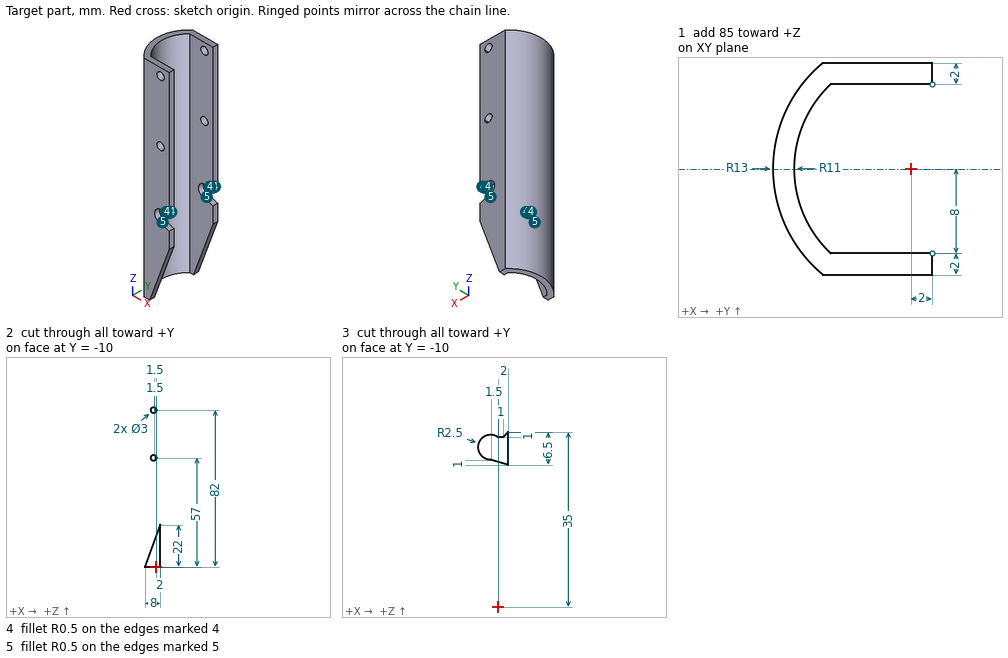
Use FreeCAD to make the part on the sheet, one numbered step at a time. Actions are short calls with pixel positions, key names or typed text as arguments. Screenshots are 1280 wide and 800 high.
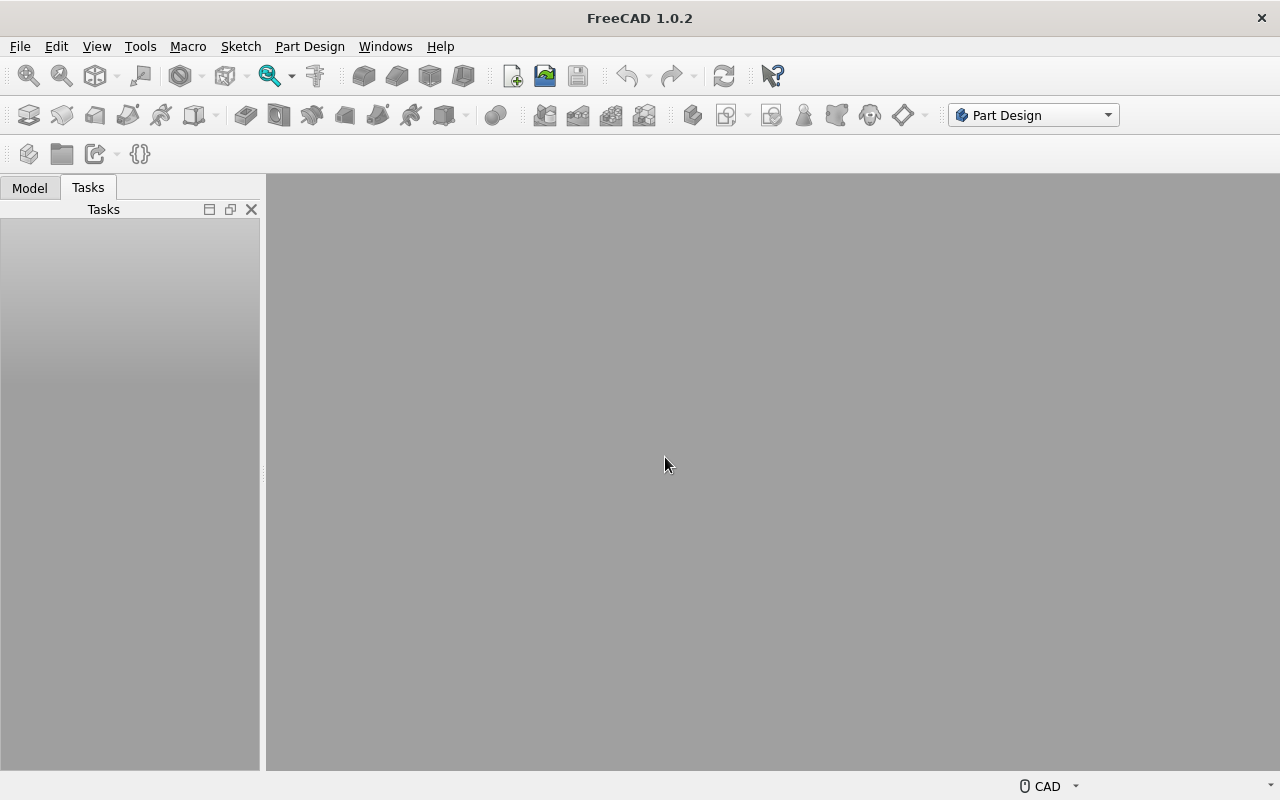
click(512, 76)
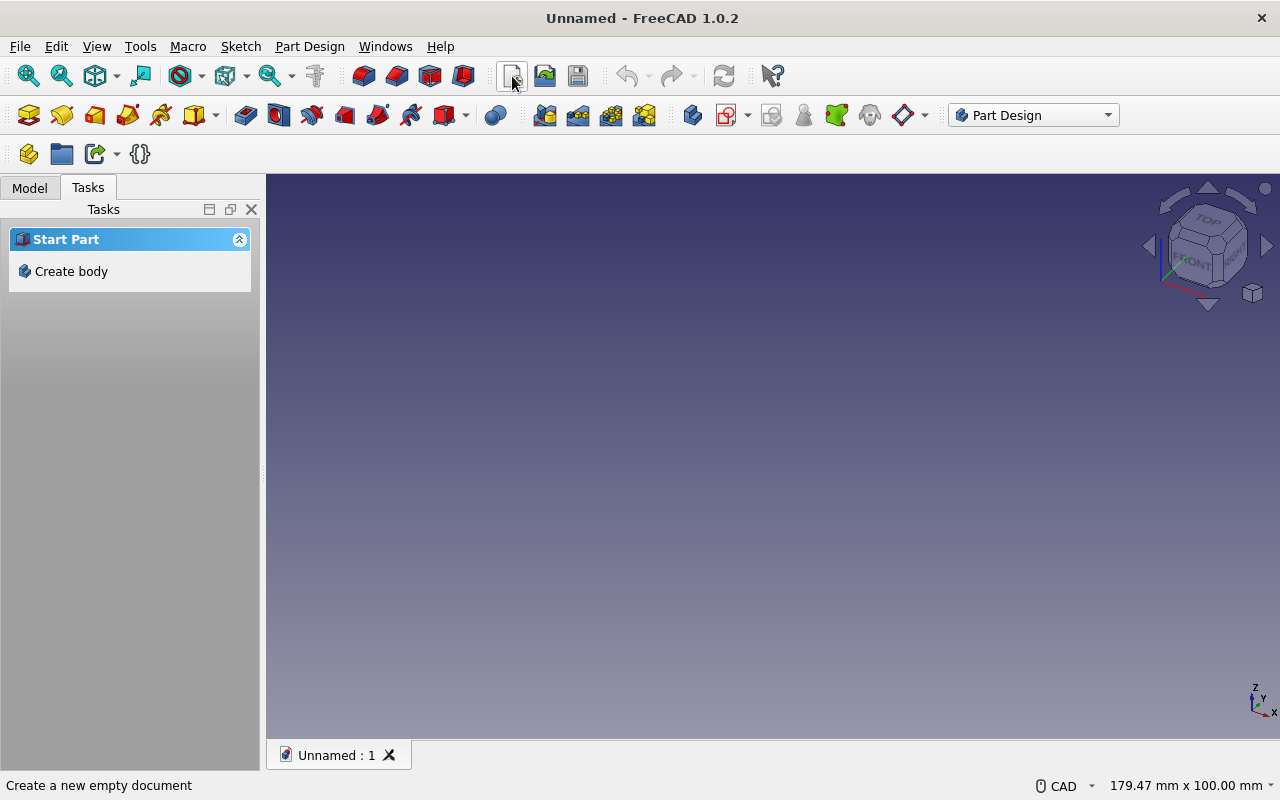
click(726, 116)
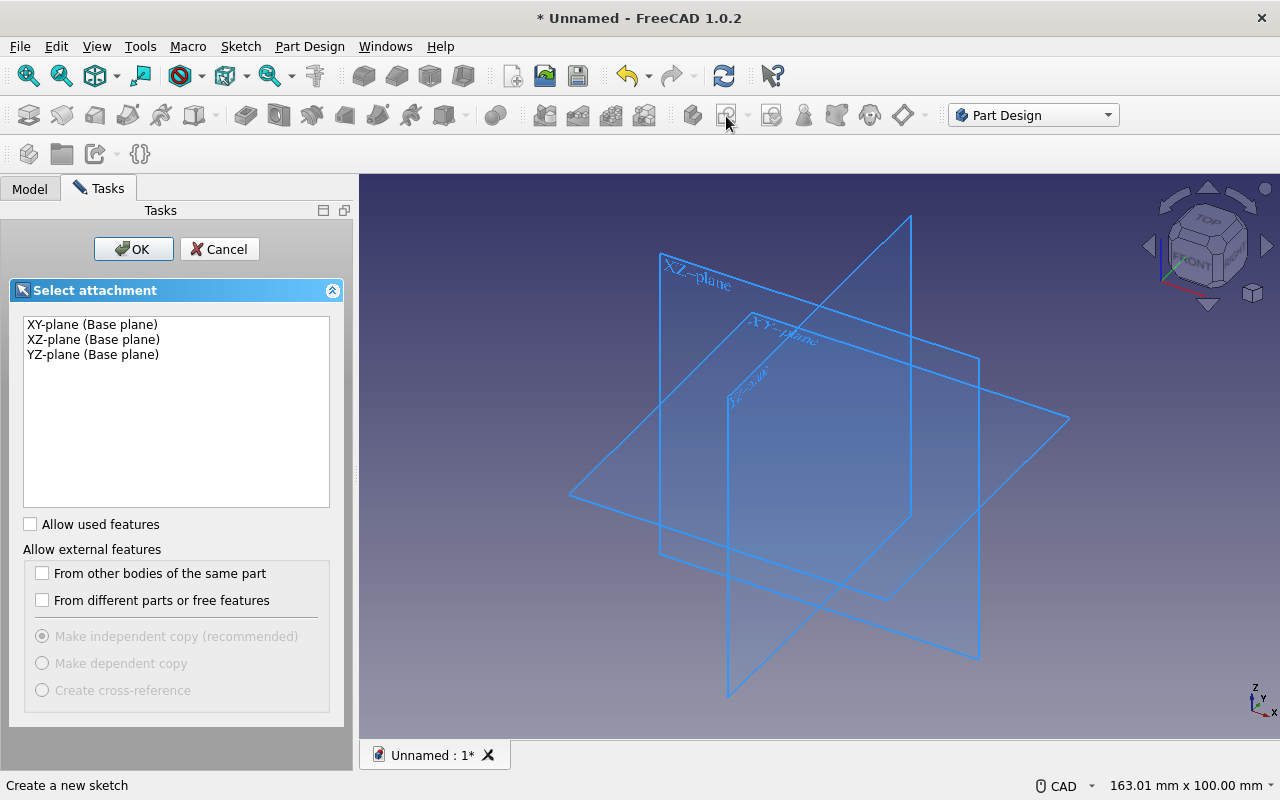
click(84, 324)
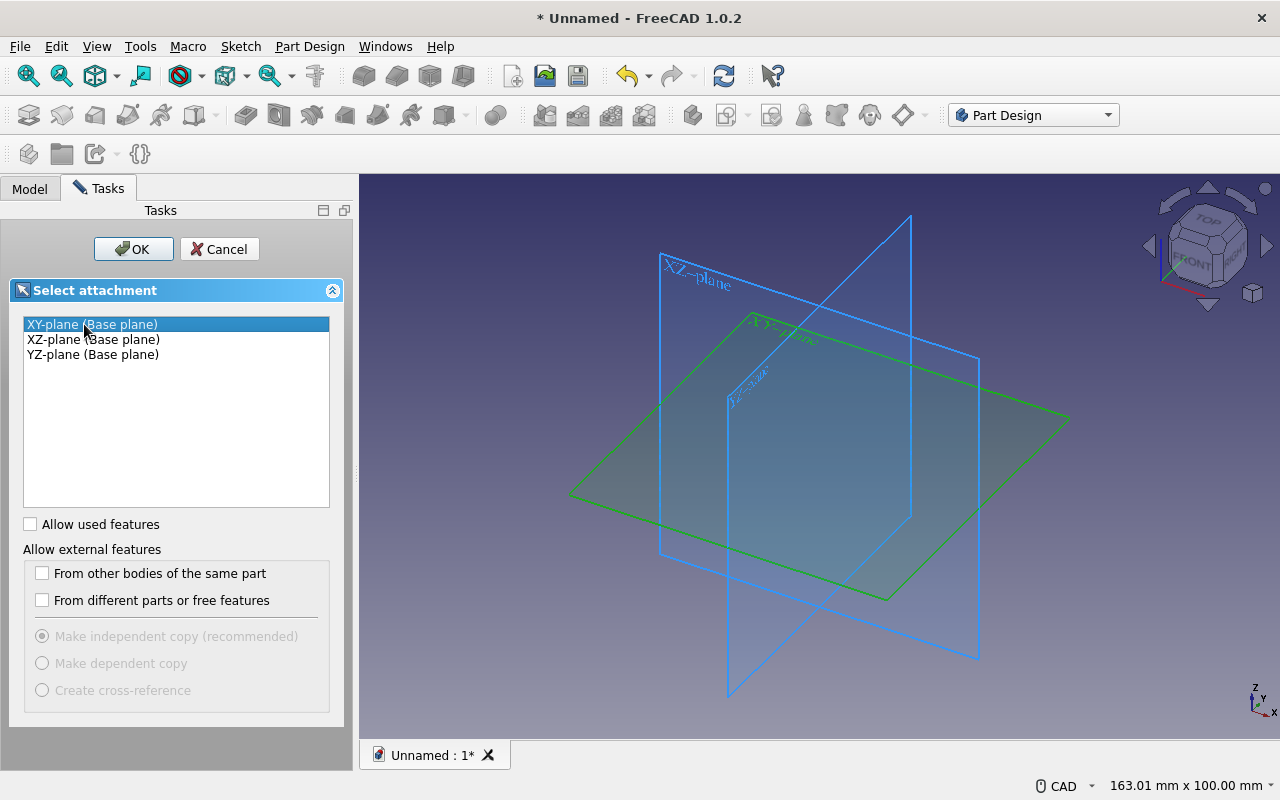
click(134, 249)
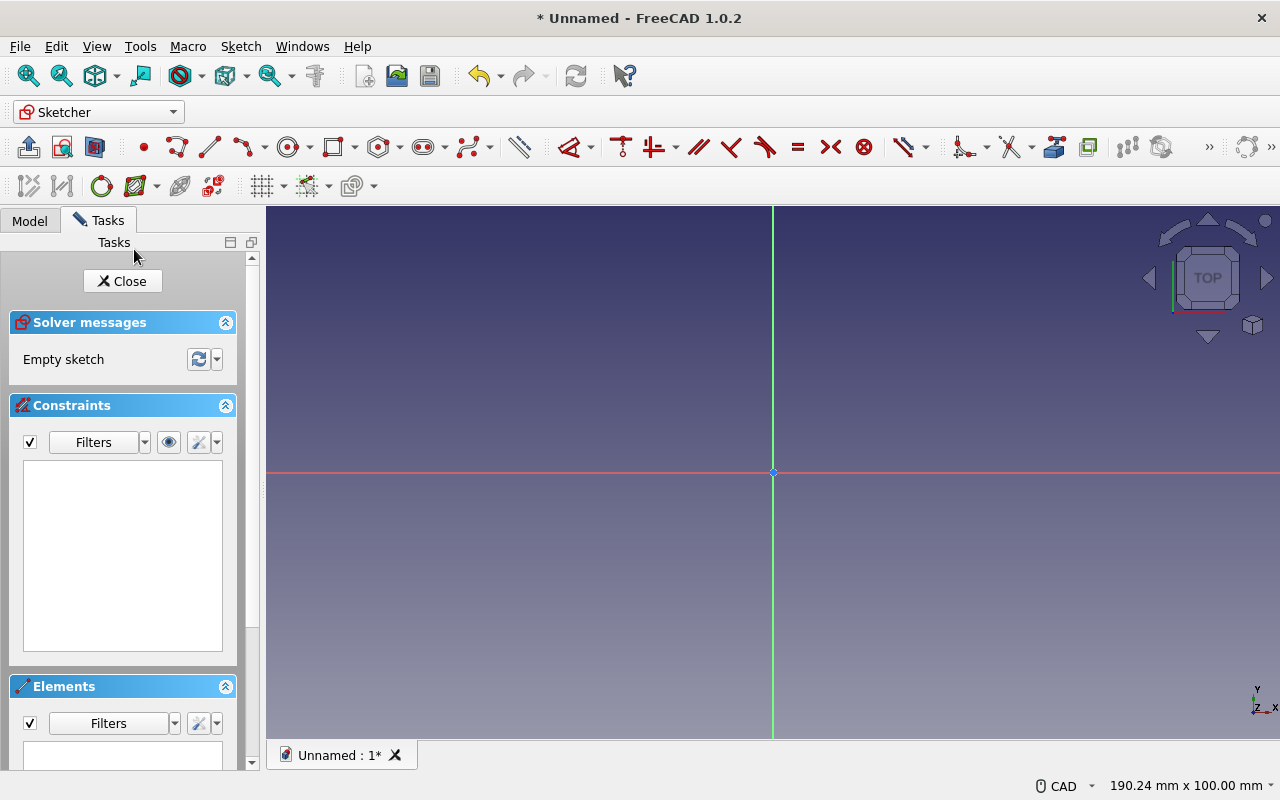
scroll(761, 472, up, 6)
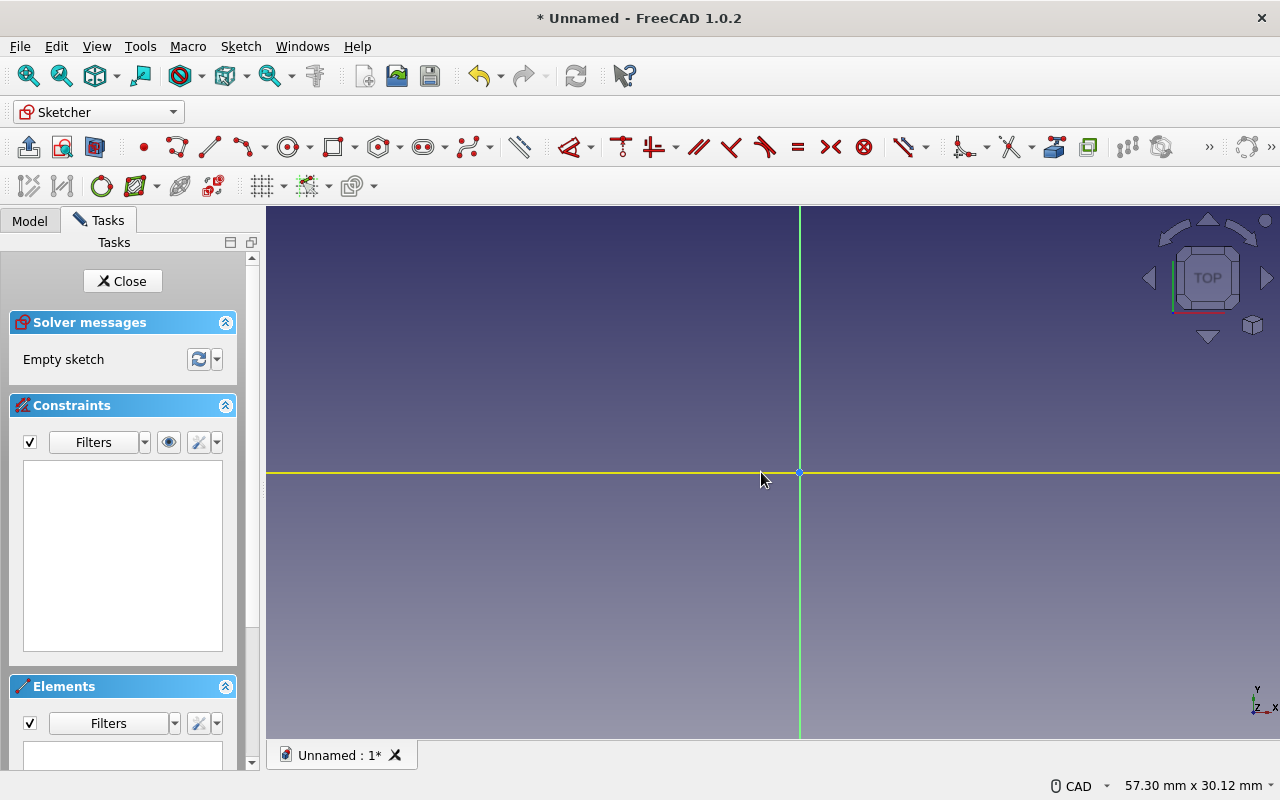
click(177, 148)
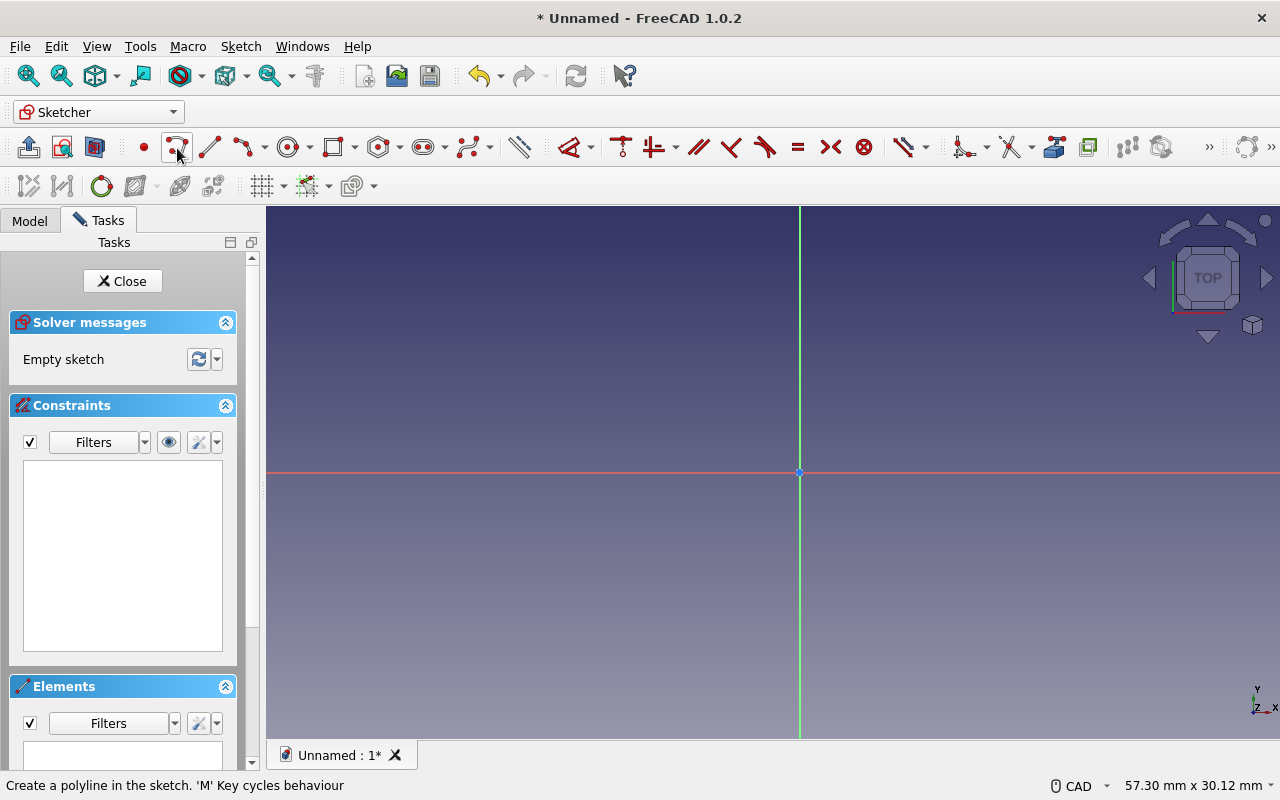
click(653, 649)
click(835, 649)
click(835, 614)
click(666, 614)
right_click(666, 614)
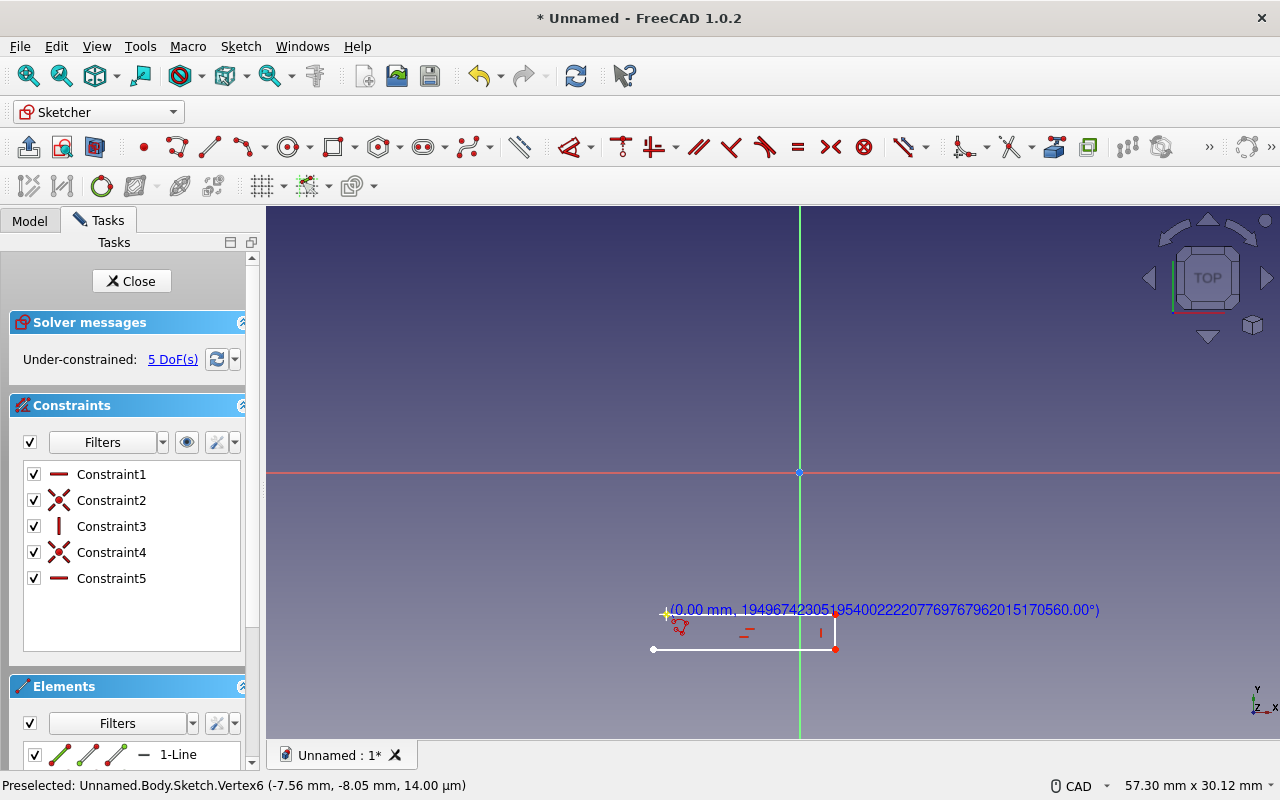
click(666, 331)
click(835, 331)
click(835, 296)
click(653, 296)
right_click(653, 296)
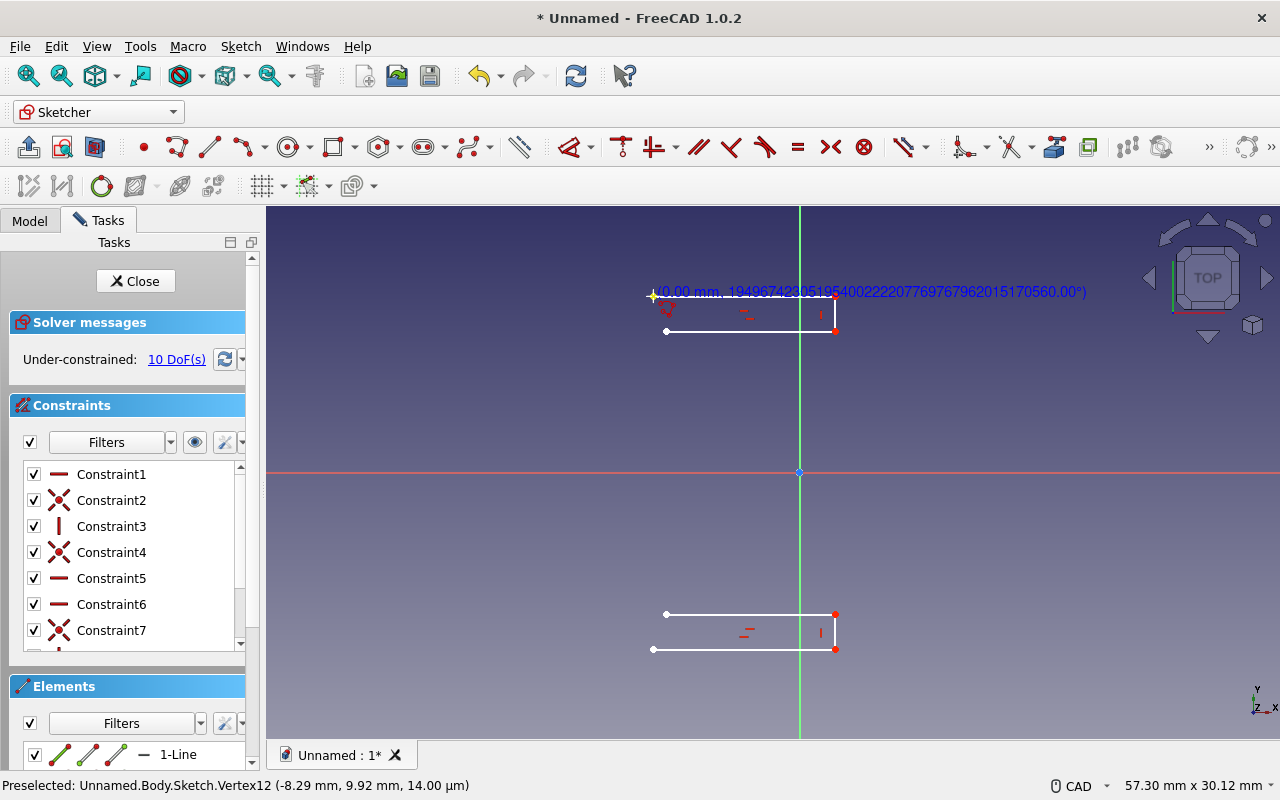
key(g)
key(3)
key(a)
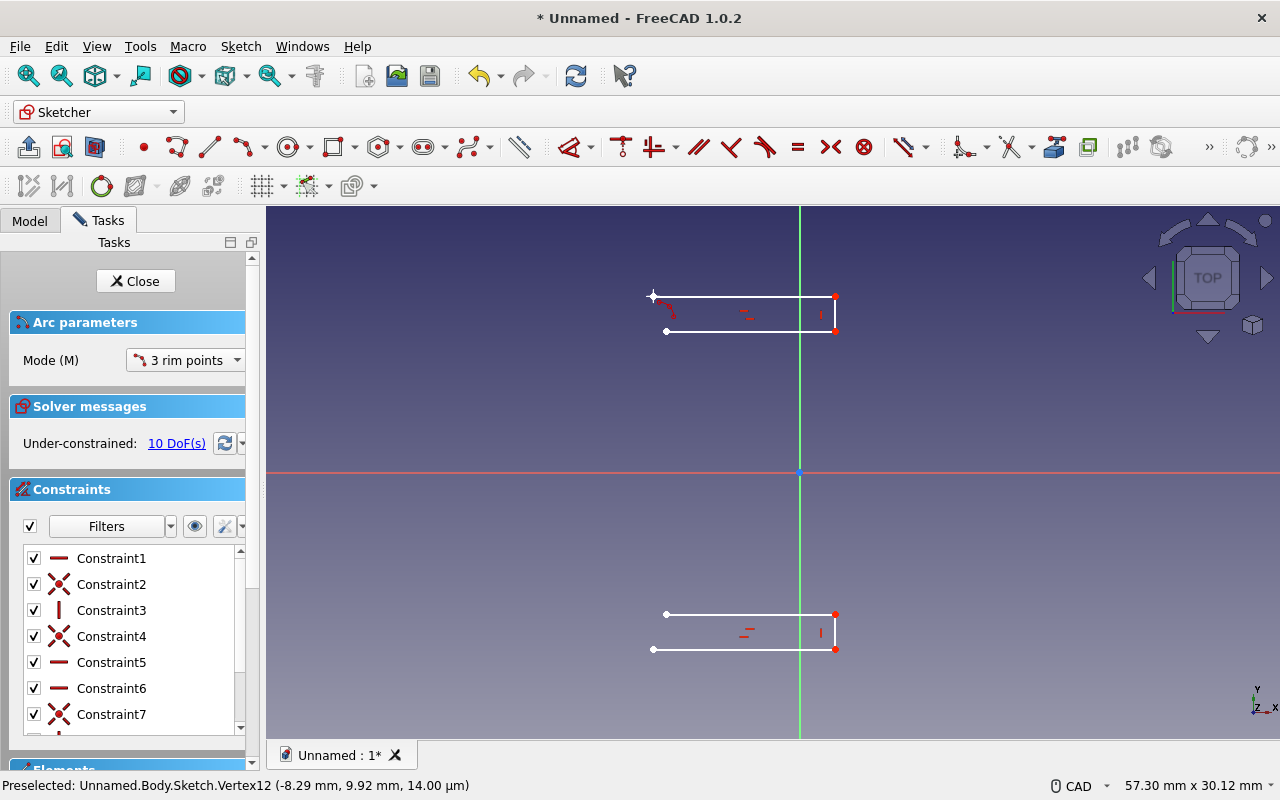
click(666, 615)
click(666, 332)
click(608, 441)